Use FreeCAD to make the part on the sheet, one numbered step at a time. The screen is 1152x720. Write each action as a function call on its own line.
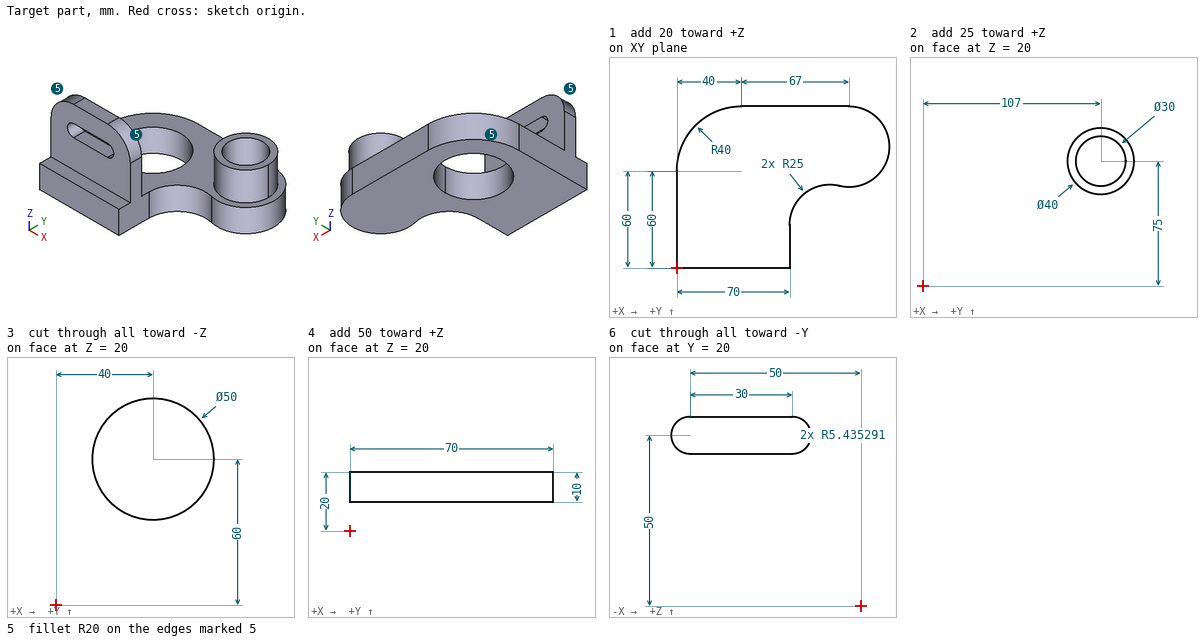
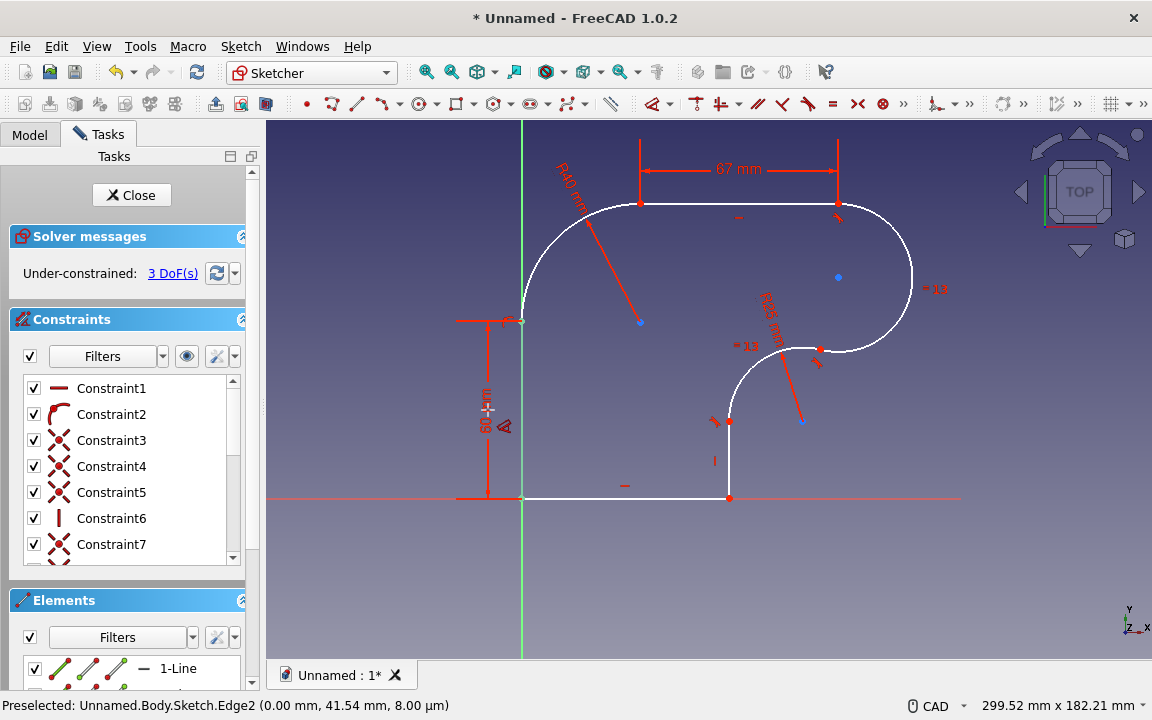
click(584, 499)
click(625, 533)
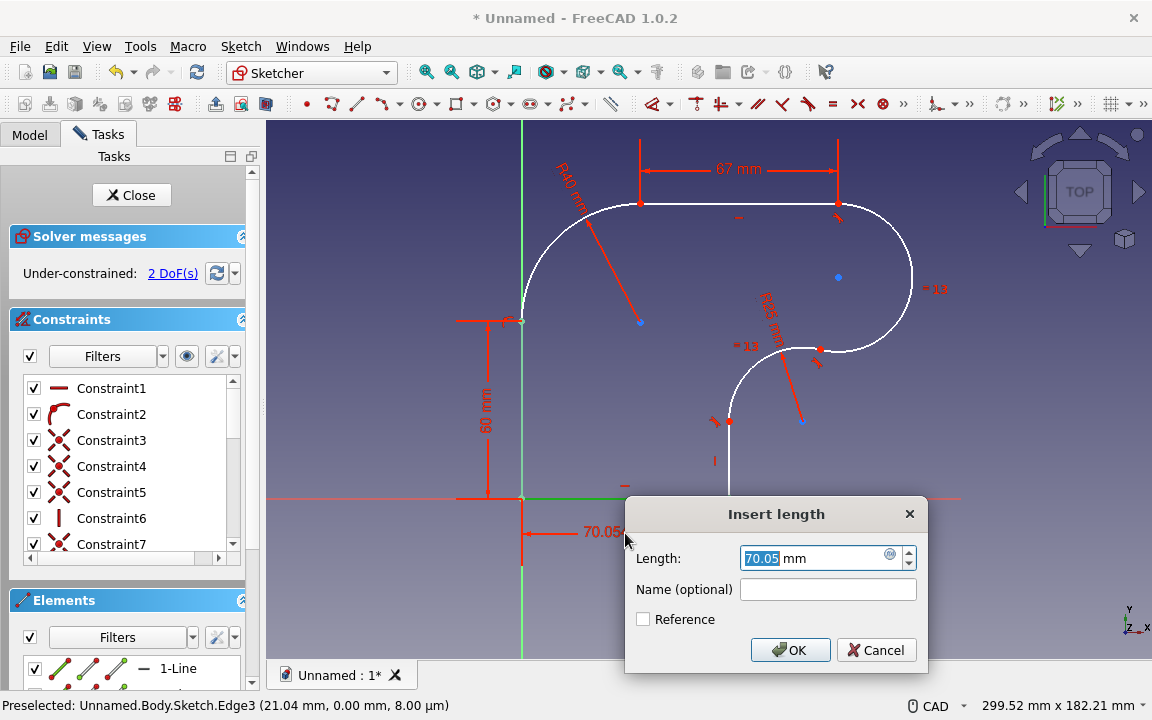
text(70)
key(Return)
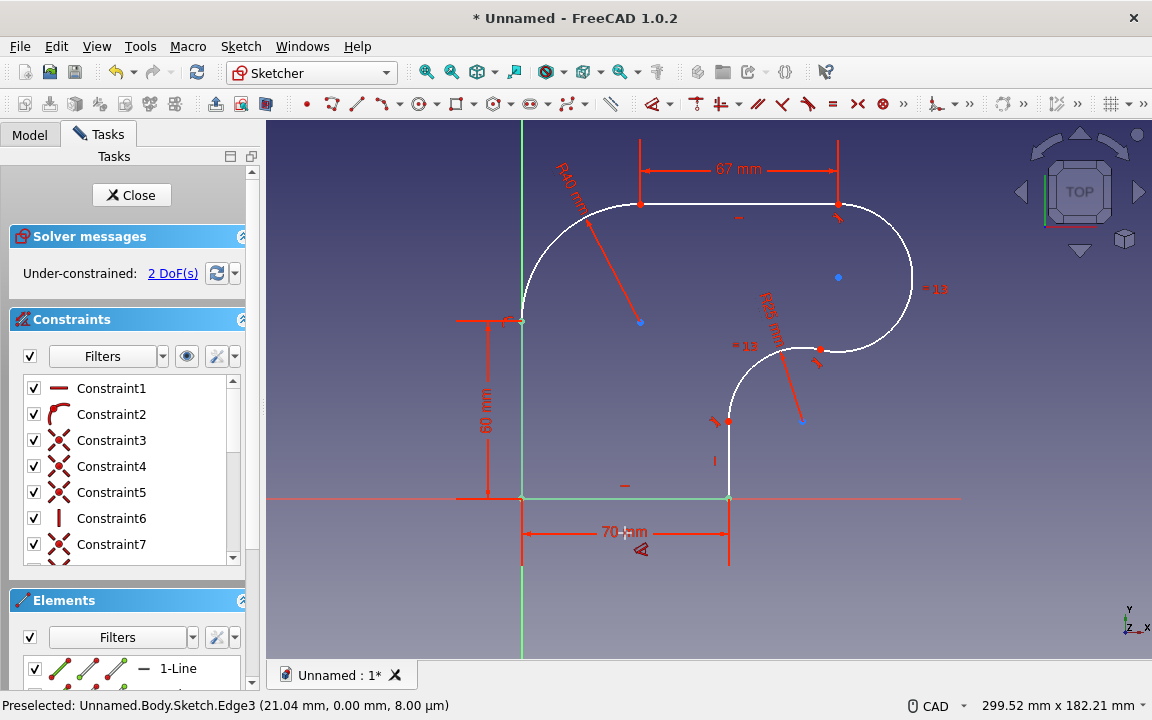
click(640, 204)
click(554, 533)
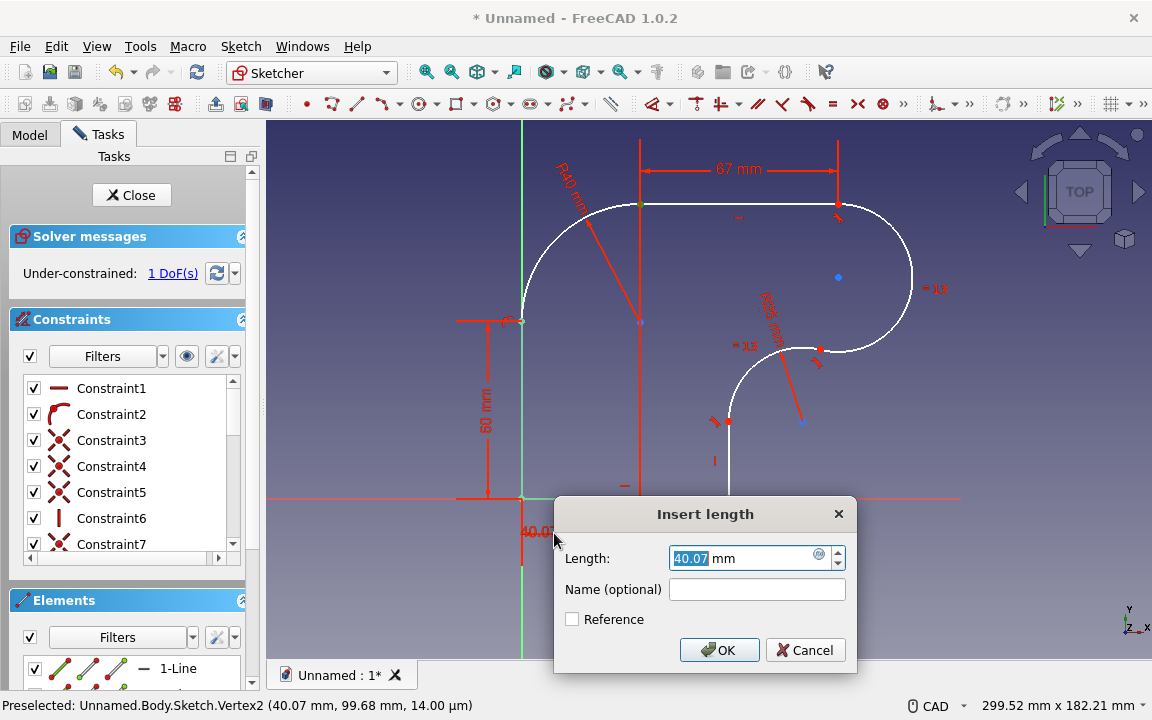
text(40)
key(Return)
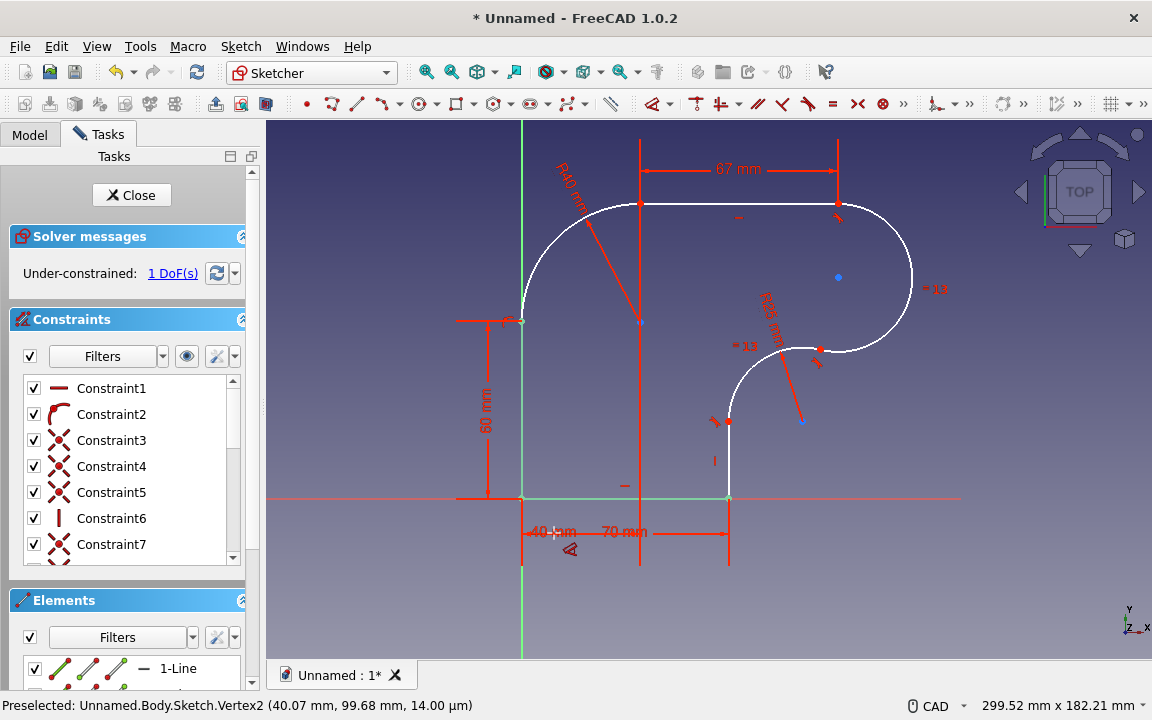
click(640, 322)
click(488, 370)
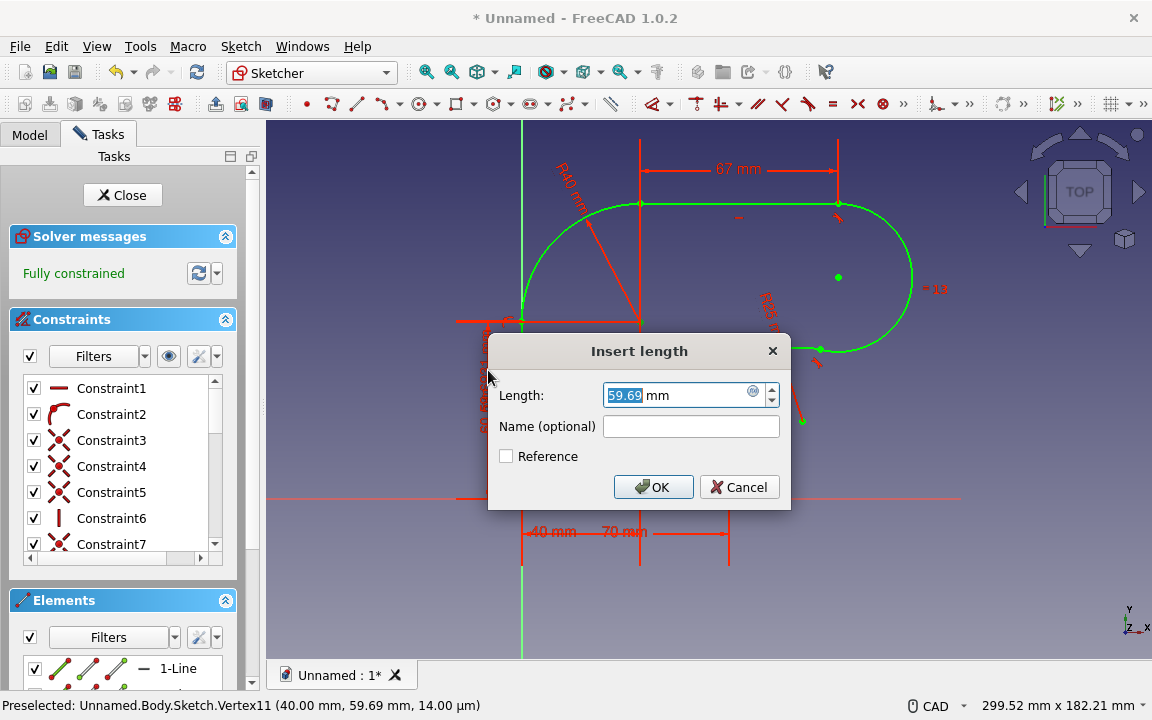
text(60)
key(Return)
key(Escape)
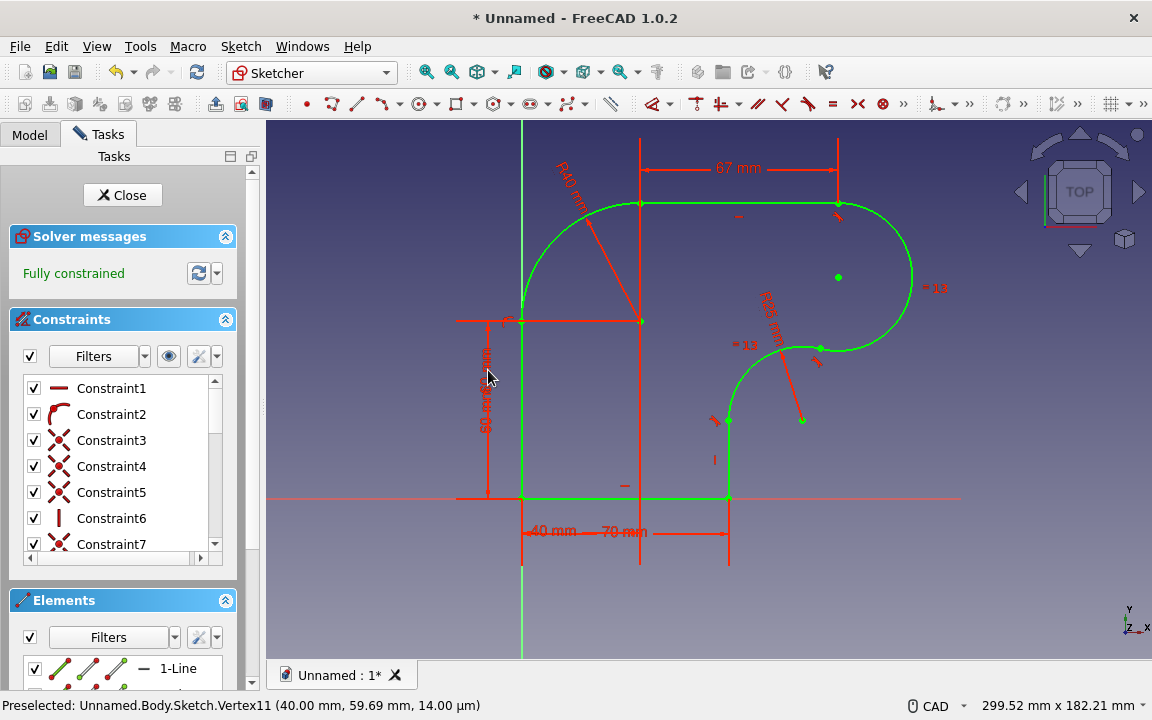
click(123, 195)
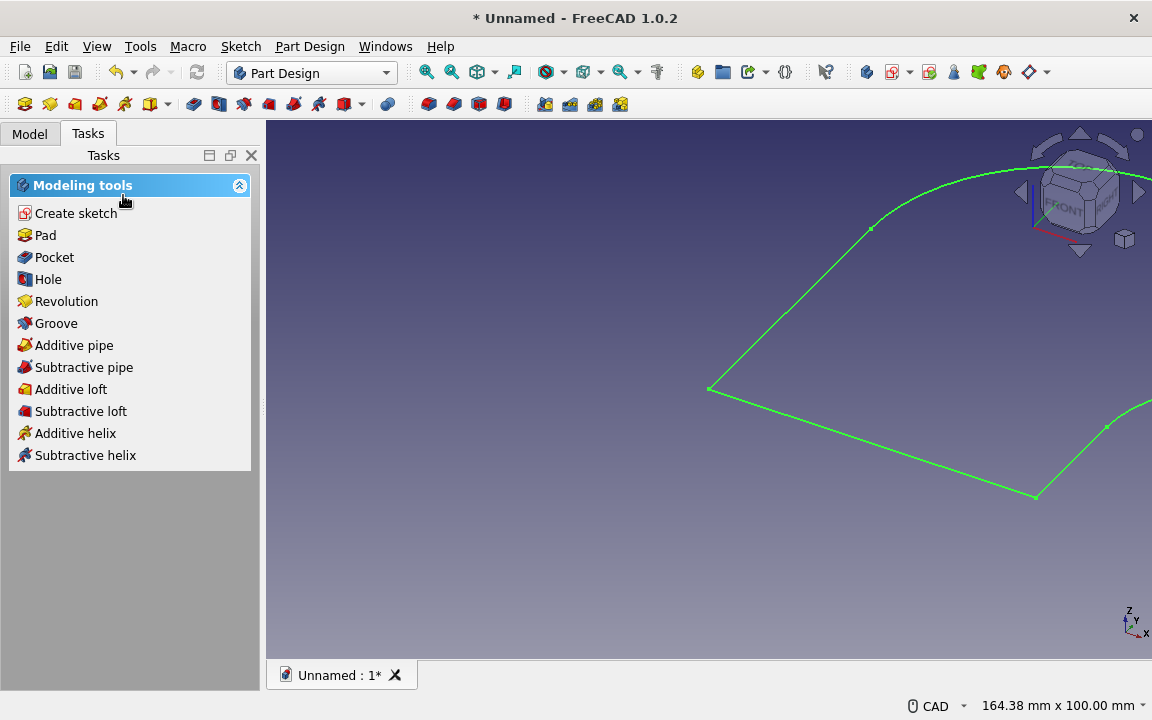
click(25, 104)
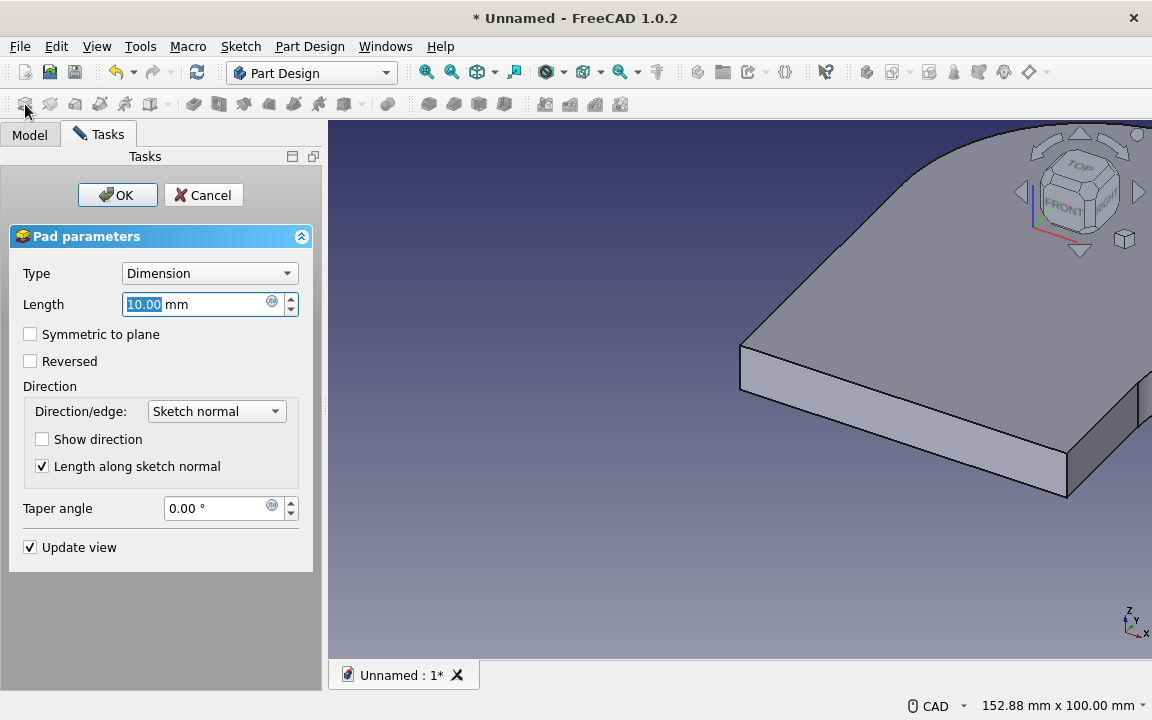
text(20)
key(Tab)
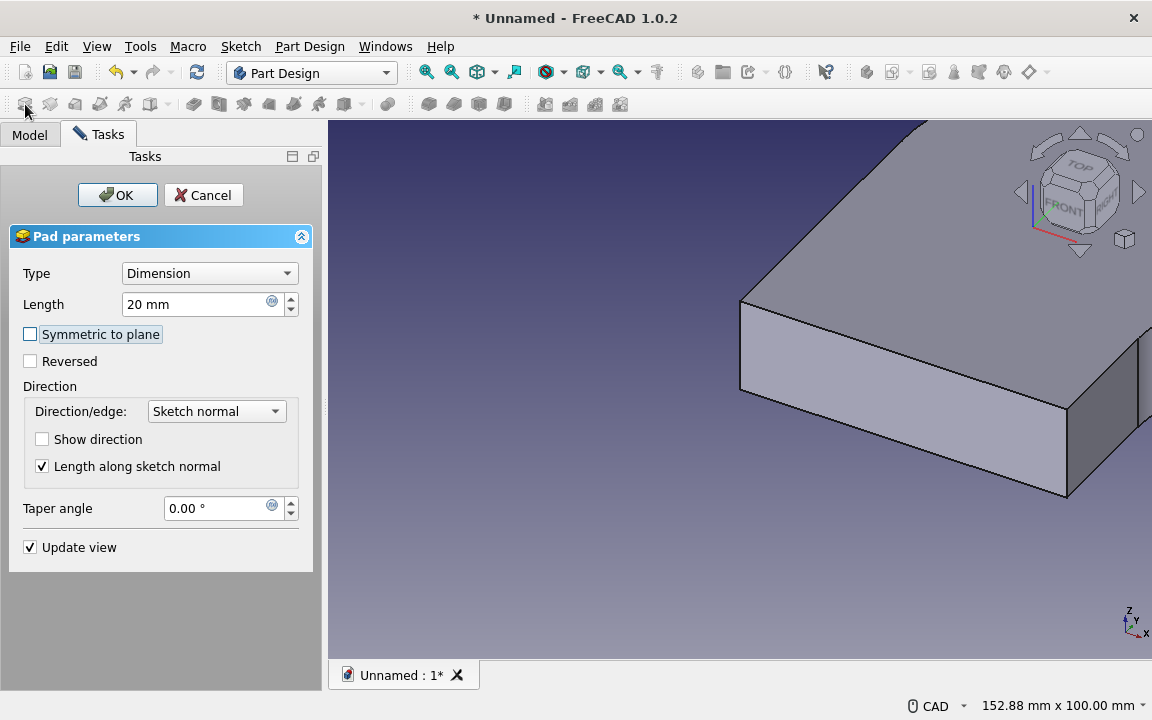
click(118, 195)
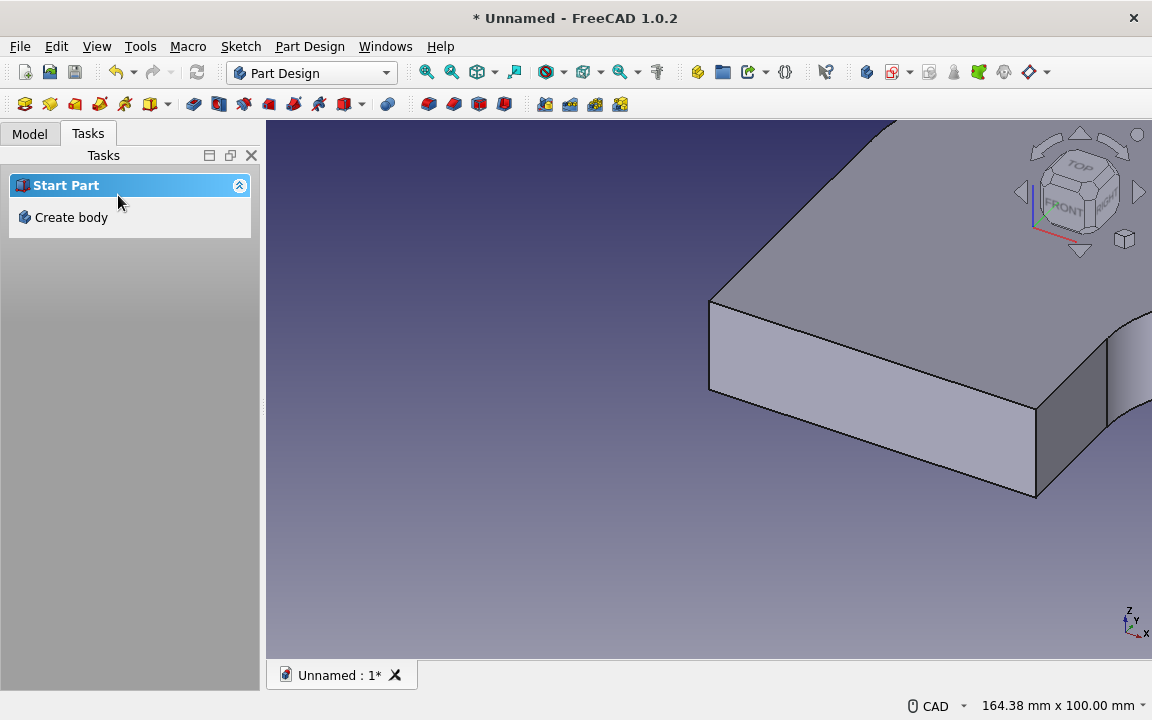
click(427, 72)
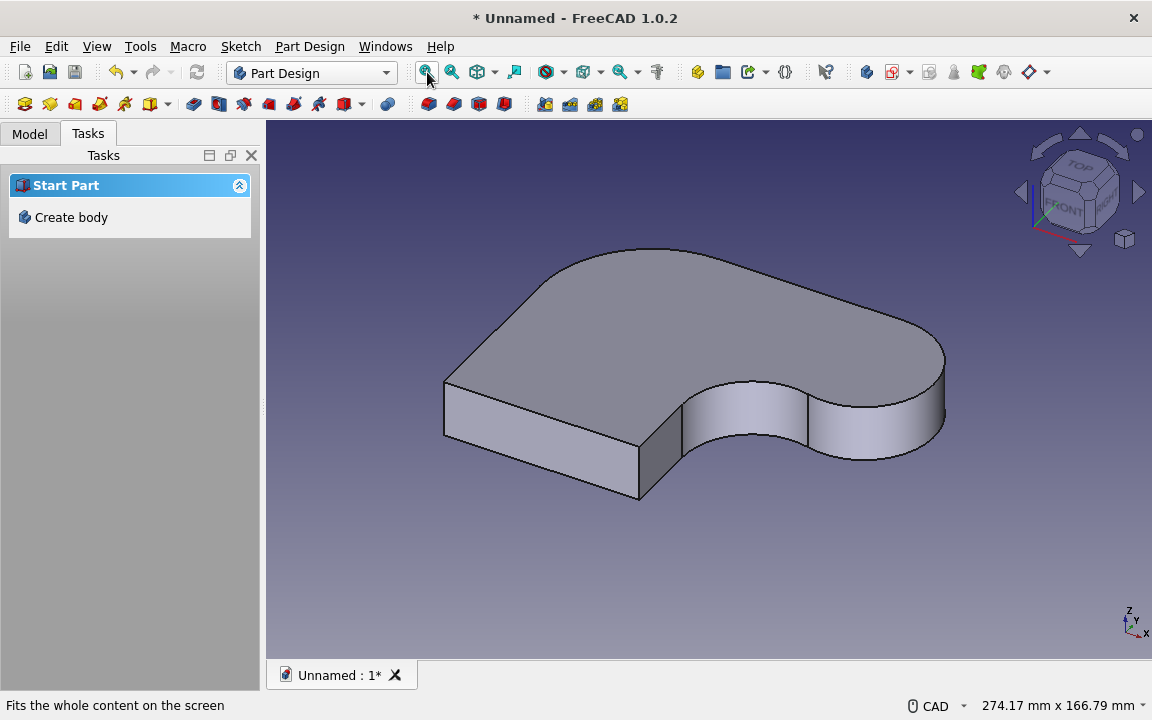
click(679, 322)